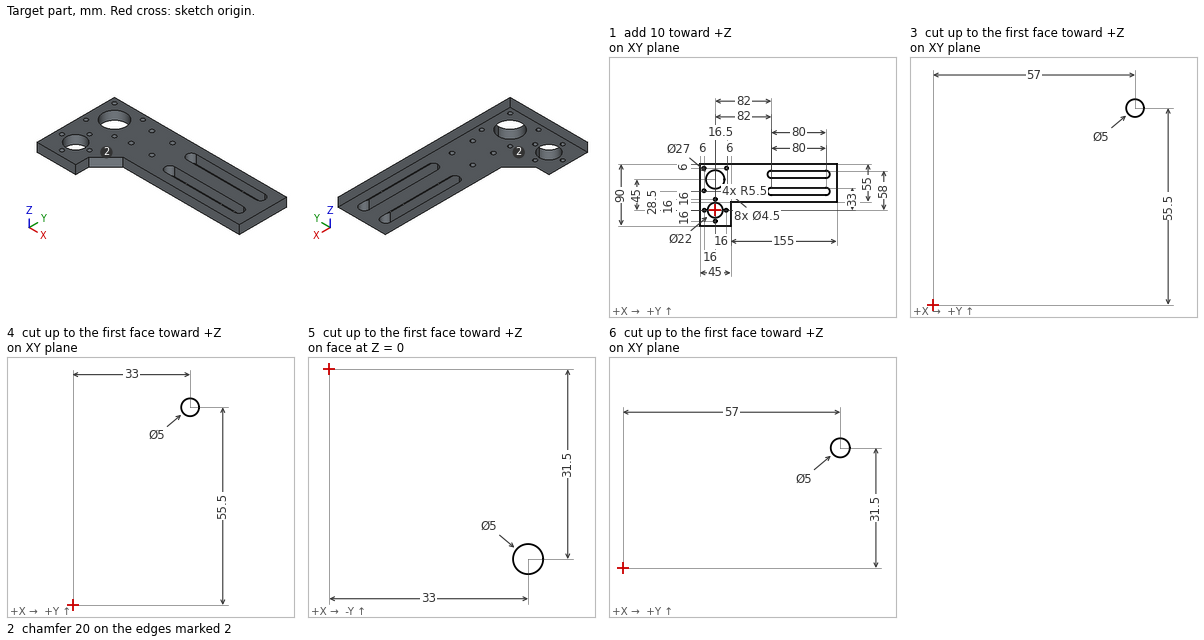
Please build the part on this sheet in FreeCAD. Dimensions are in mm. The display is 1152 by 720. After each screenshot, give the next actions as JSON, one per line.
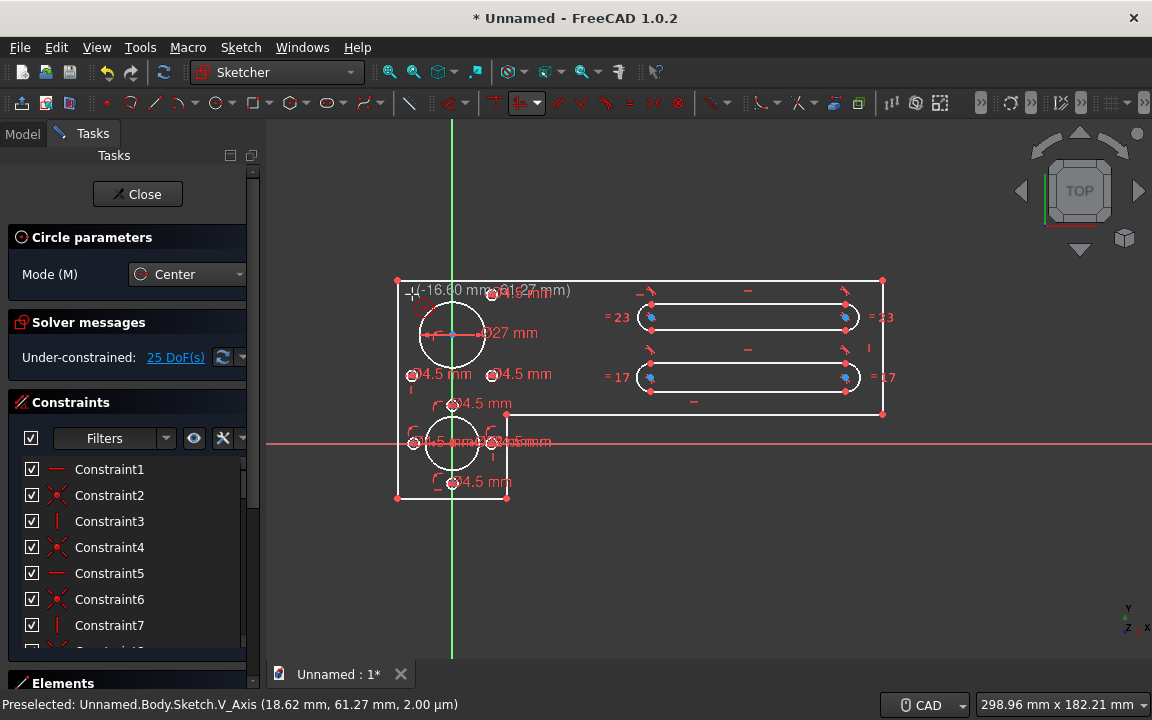
{"action": "left_click", "coordinate": [412, 294]}
{"action": "mouse_move", "coordinate": [416, 298]}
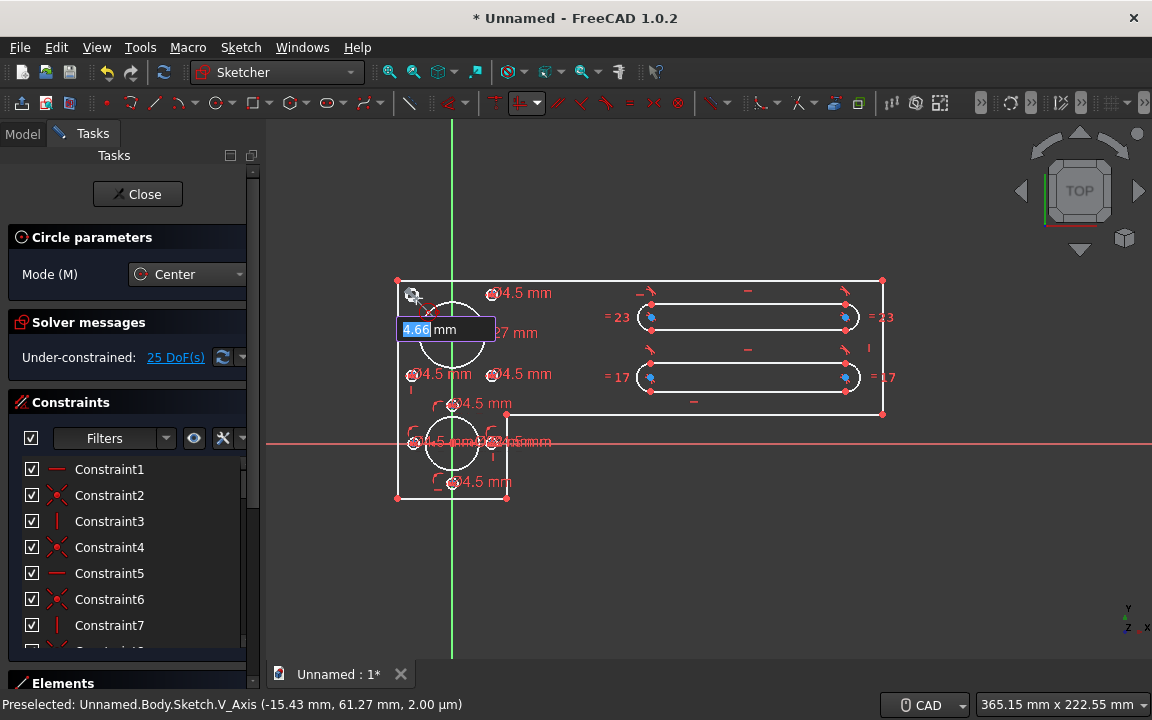
{"action": "type", "text": "4.5"}
{"action": "key", "text": "Return"}
{"action": "key", "text": "Escape"}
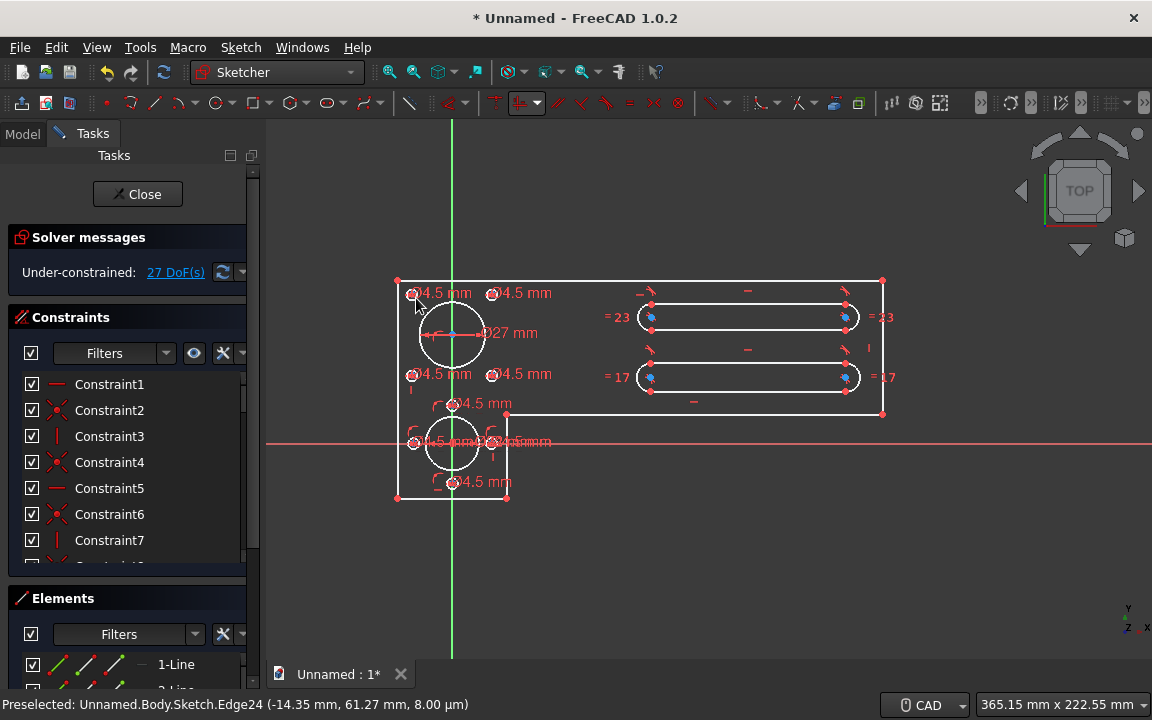
{"action": "left_click", "coordinate": [639, 369]}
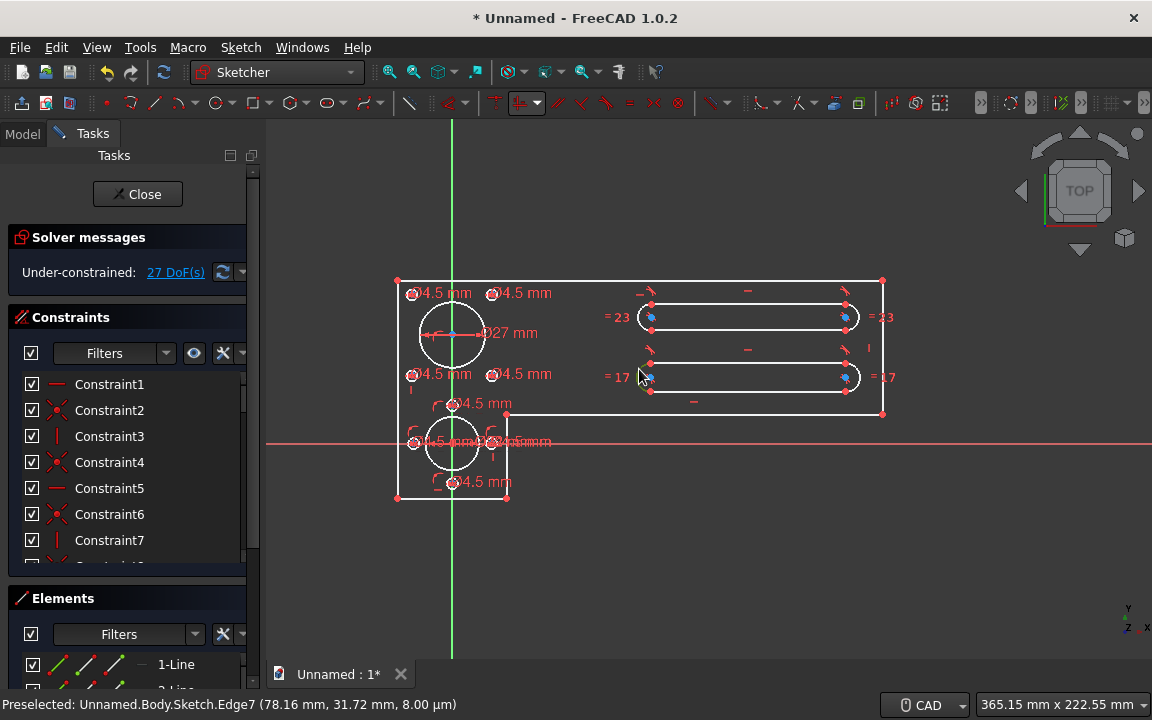
{"action": "left_click", "coordinate": [640, 310]}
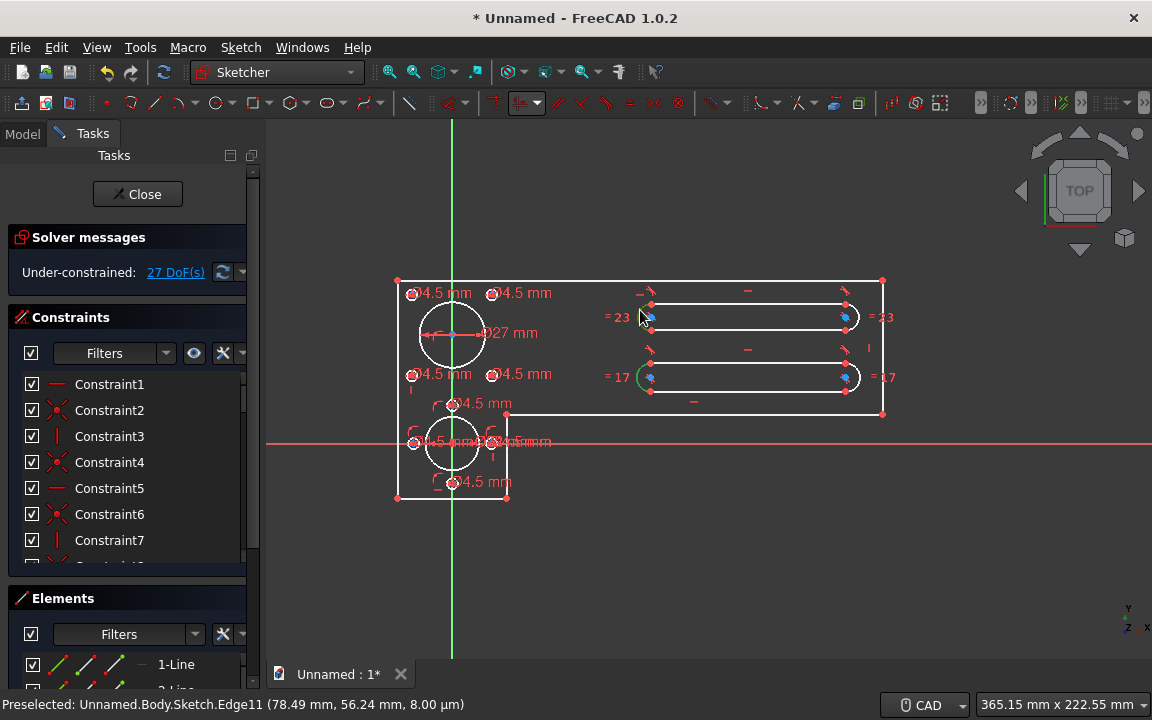
{"action": "key", "text": "e"}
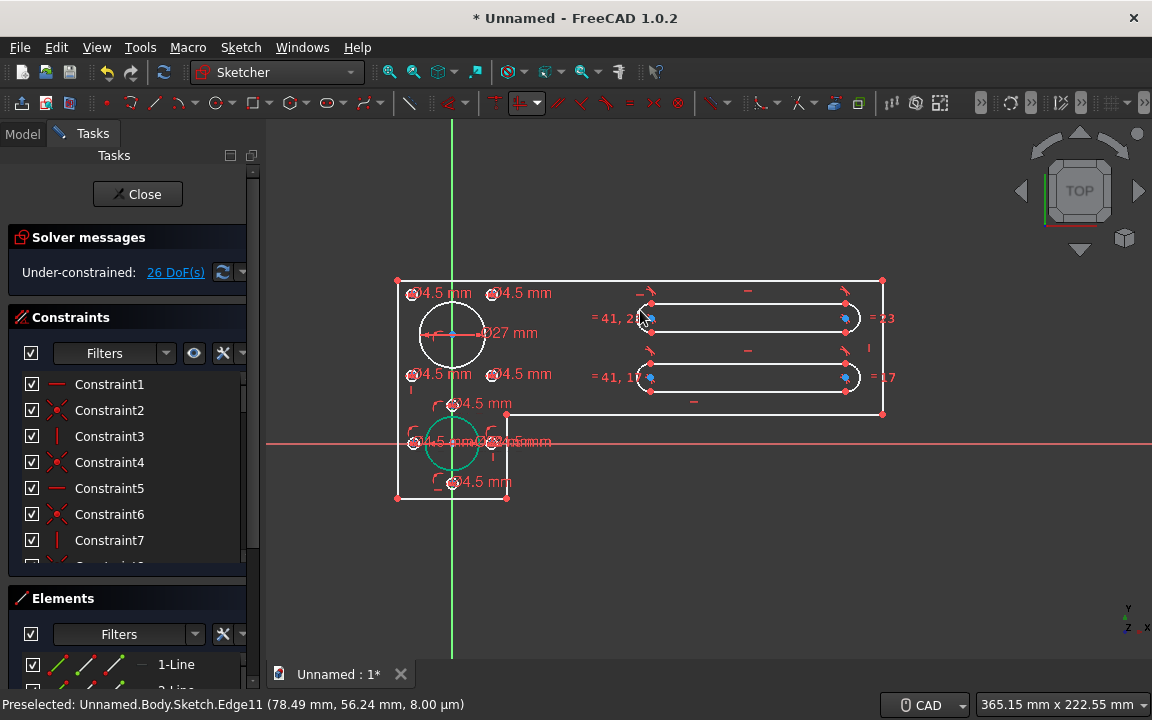
{"action": "left_click", "coordinate": [492, 376]}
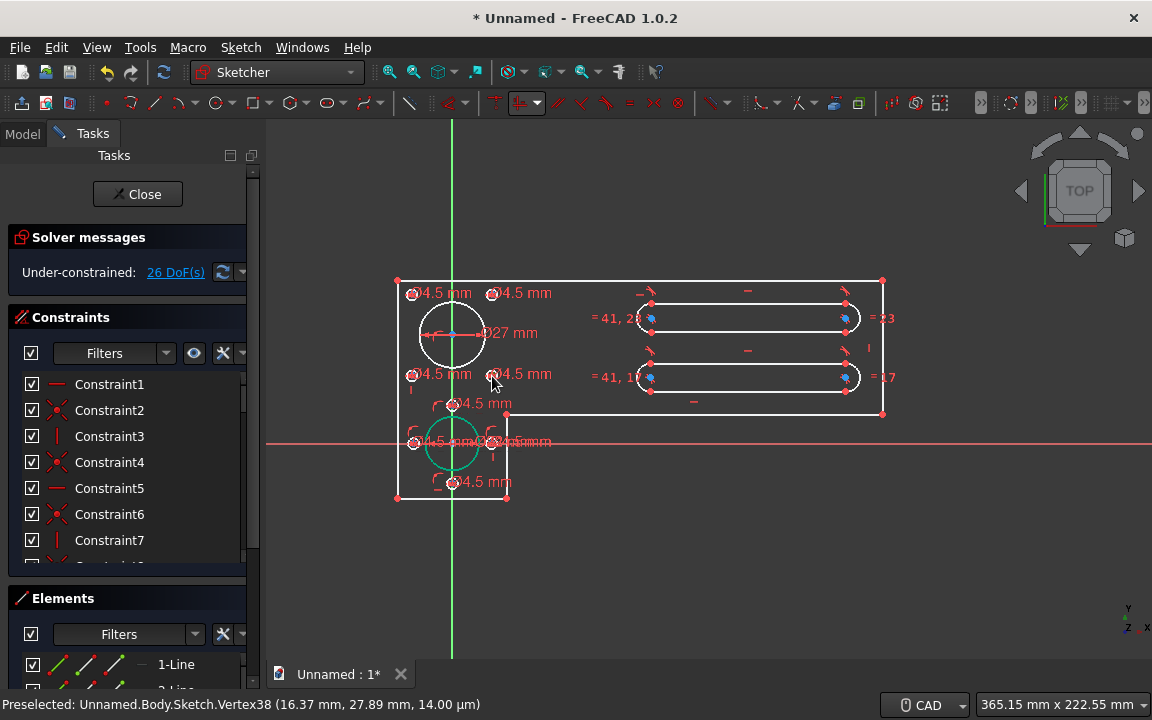
{"action": "left_click", "coordinate": [412, 376]}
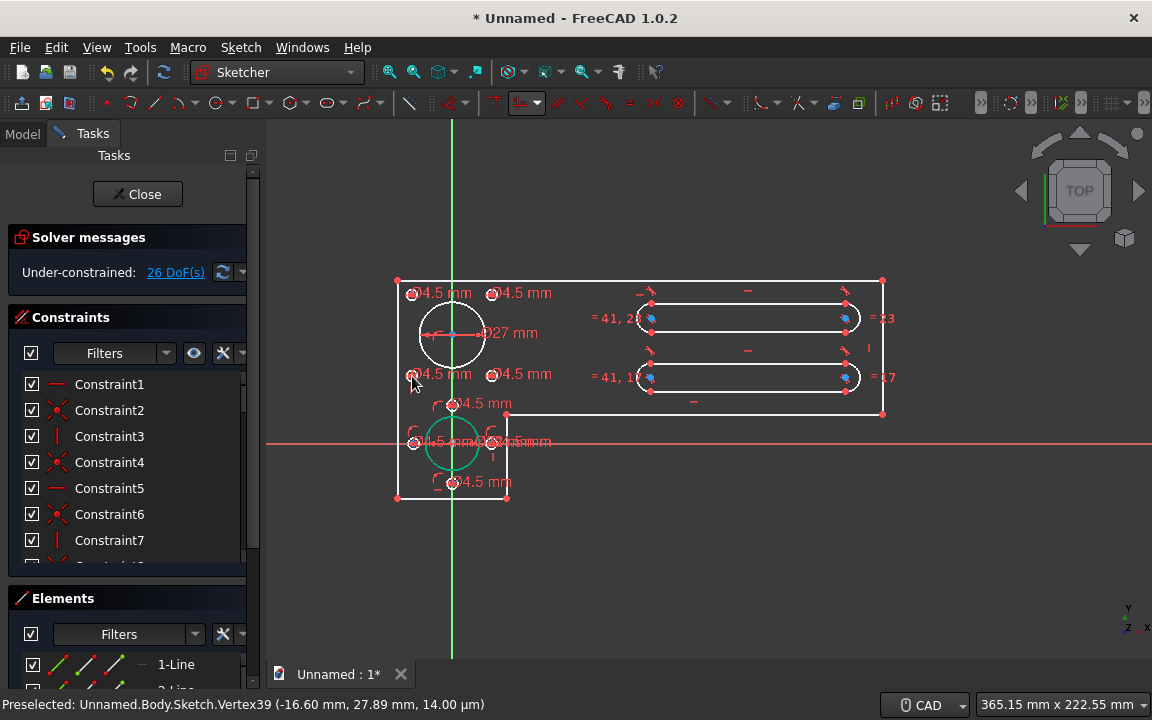
{"action": "key", "text": "h"}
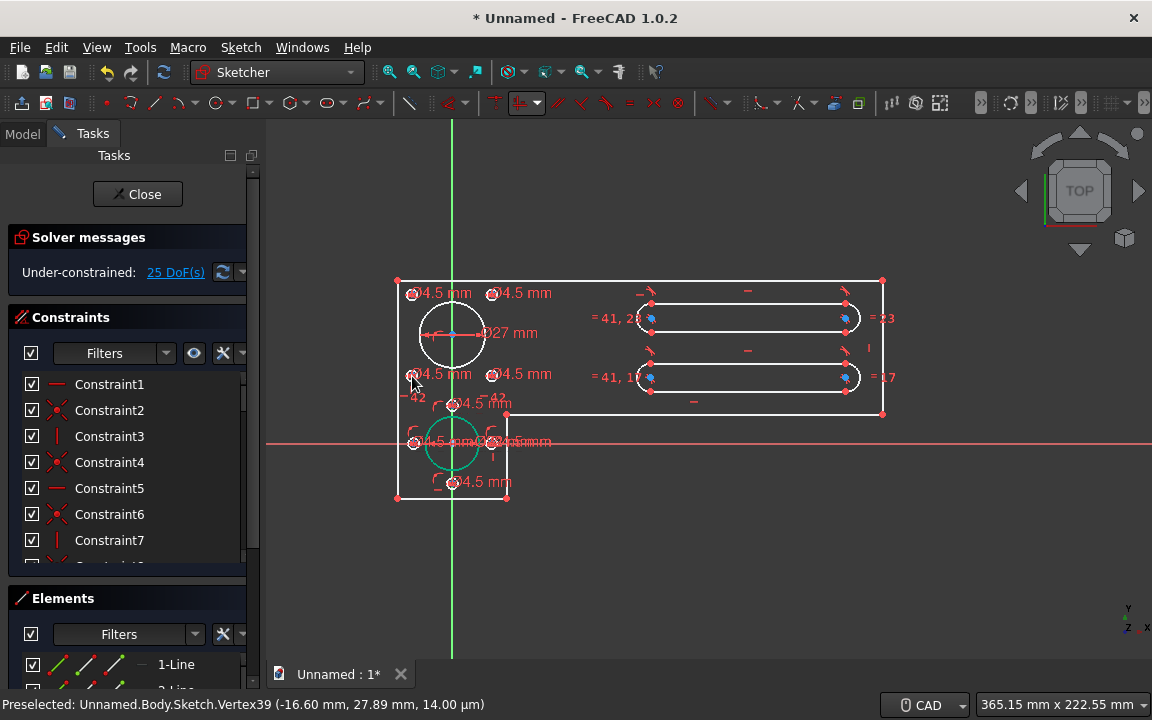
{"action": "left_click", "coordinate": [492, 376]}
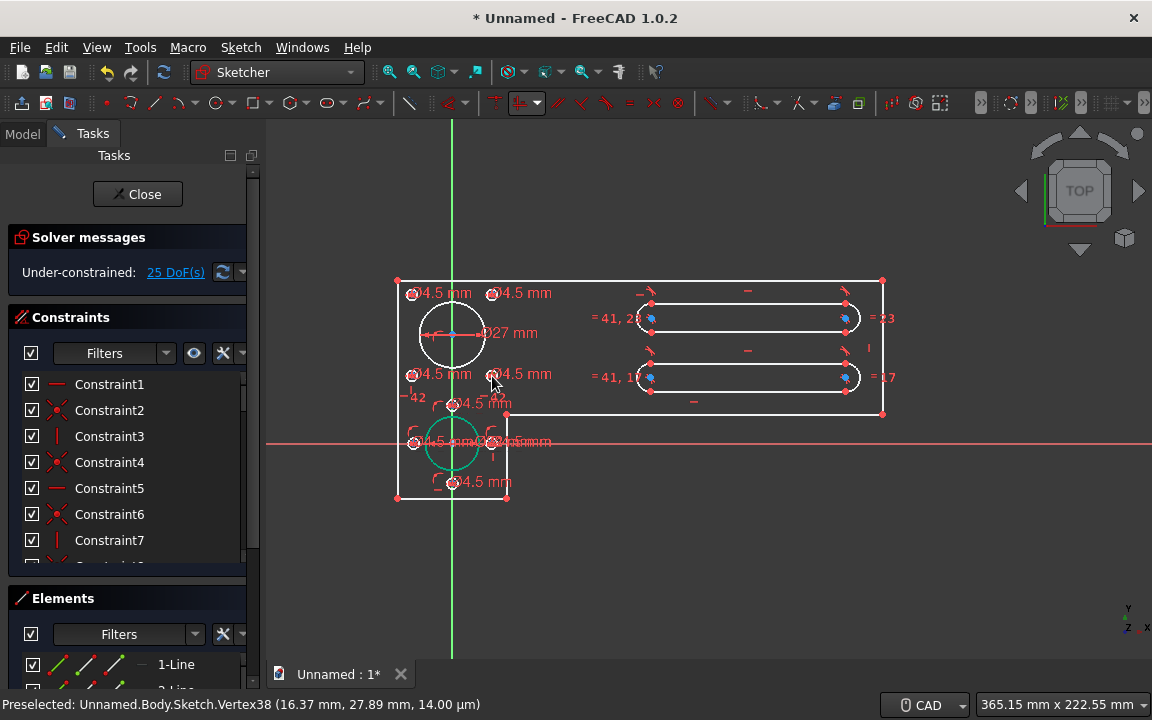
{"action": "left_click", "coordinate": [492, 295]}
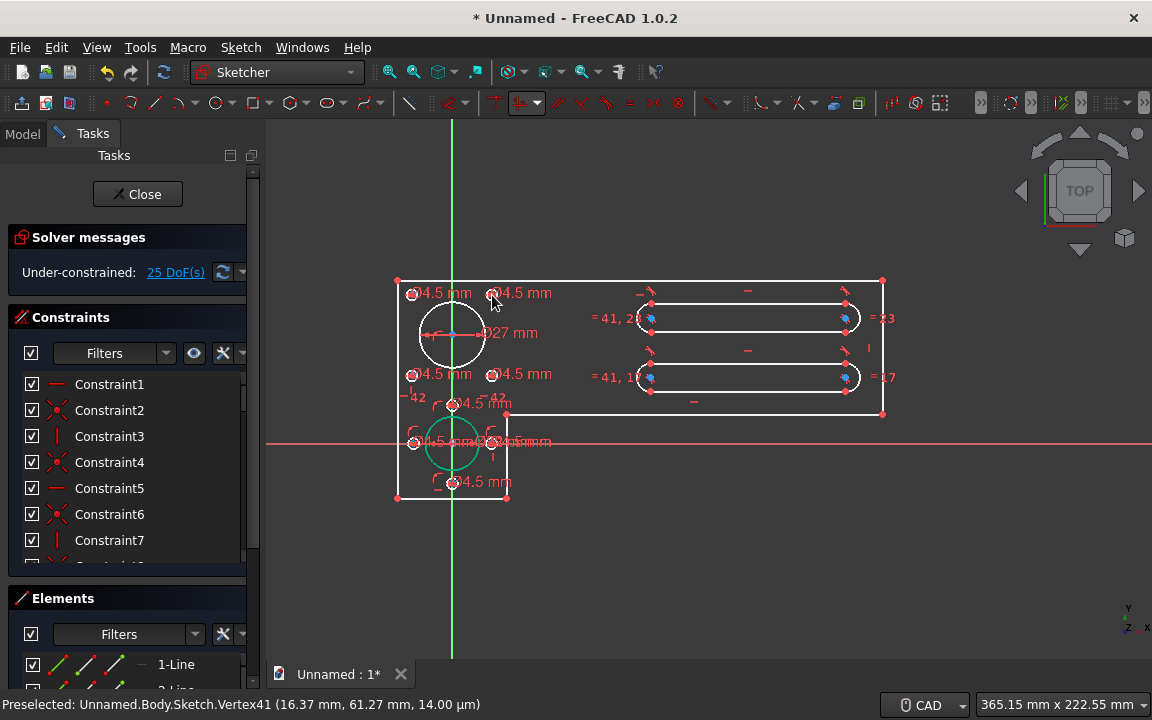
{"action": "key", "text": "v"}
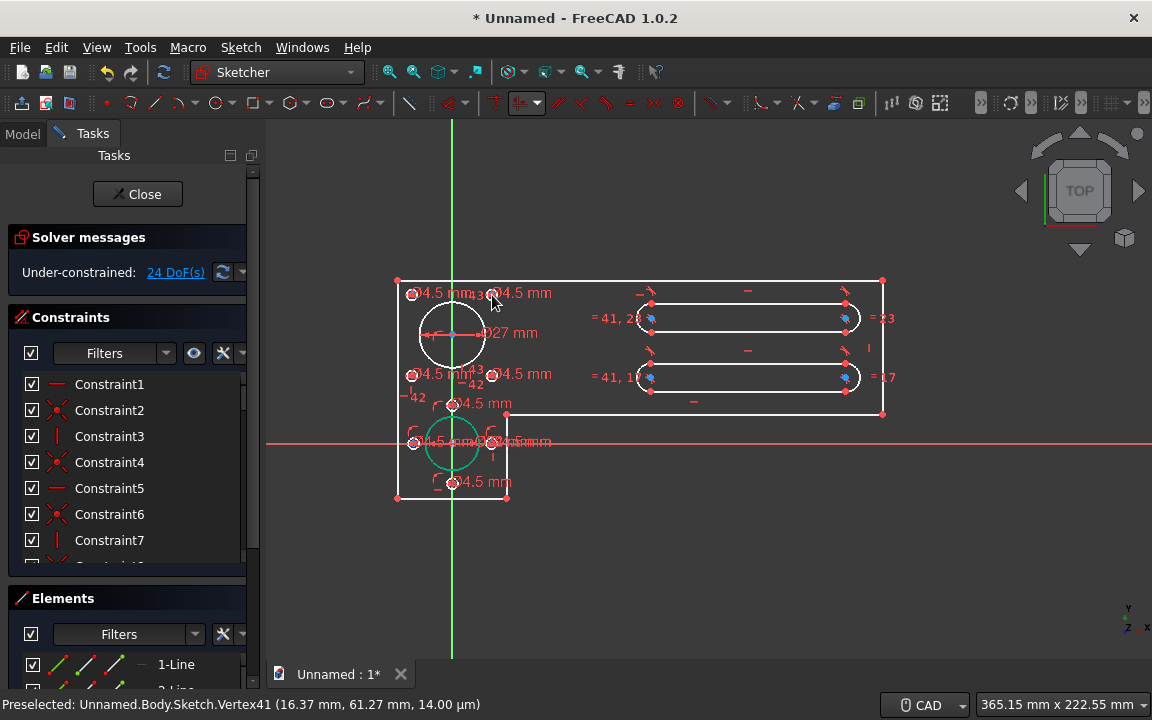
{"action": "left_click", "coordinate": [412, 376]}